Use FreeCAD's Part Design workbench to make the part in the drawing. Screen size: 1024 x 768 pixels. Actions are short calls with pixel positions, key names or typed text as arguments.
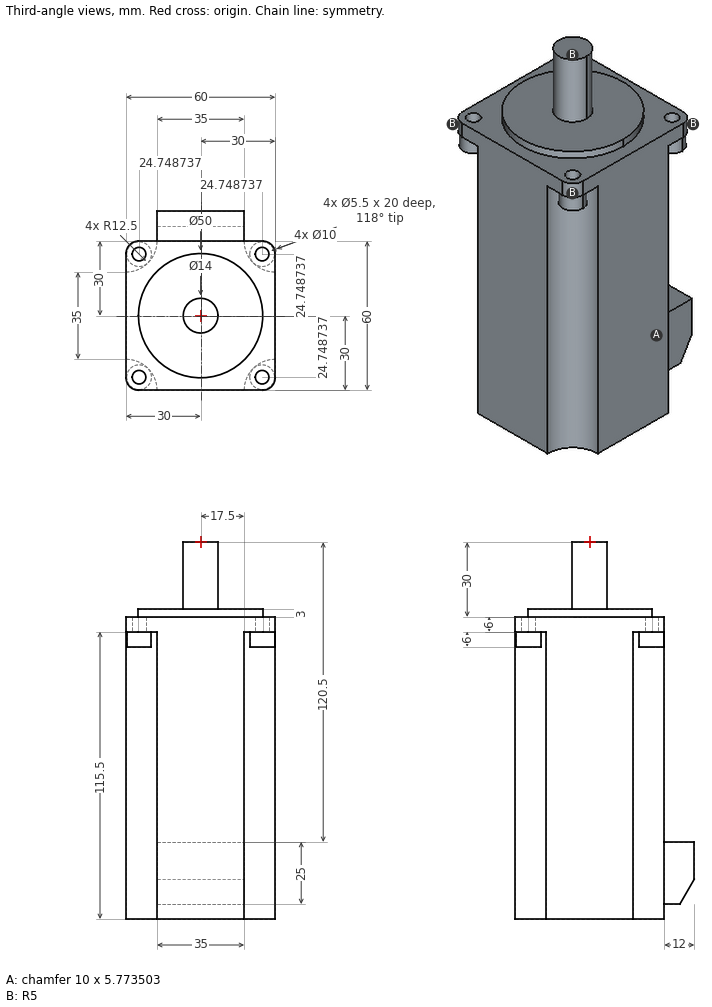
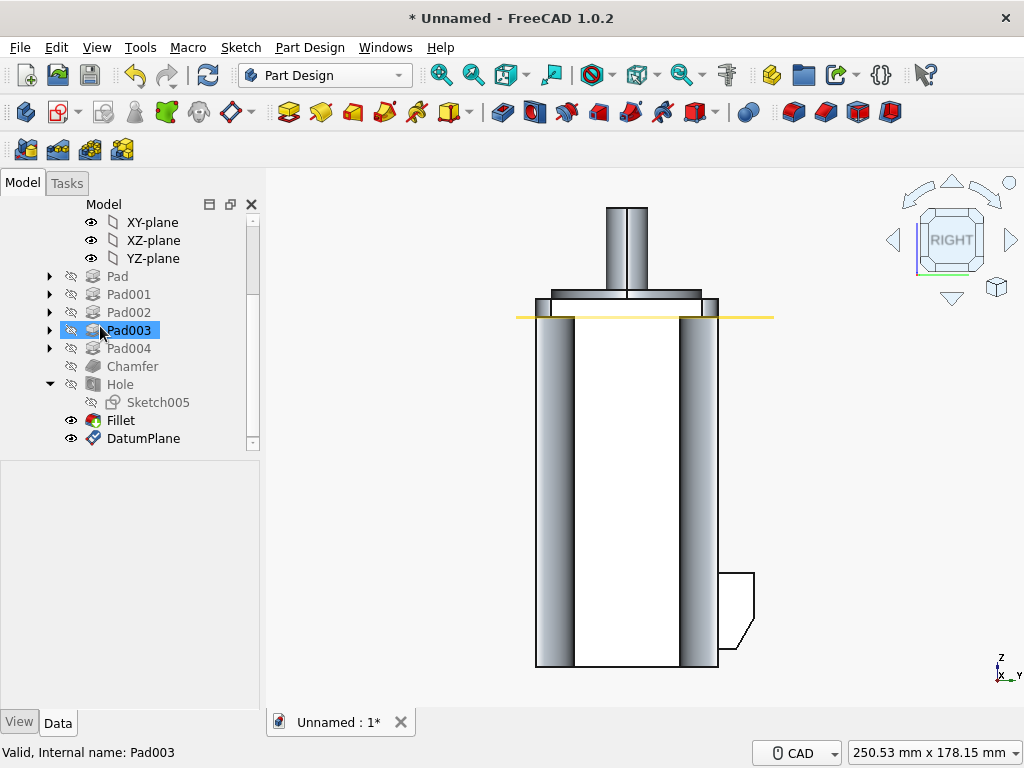
click(116, 438)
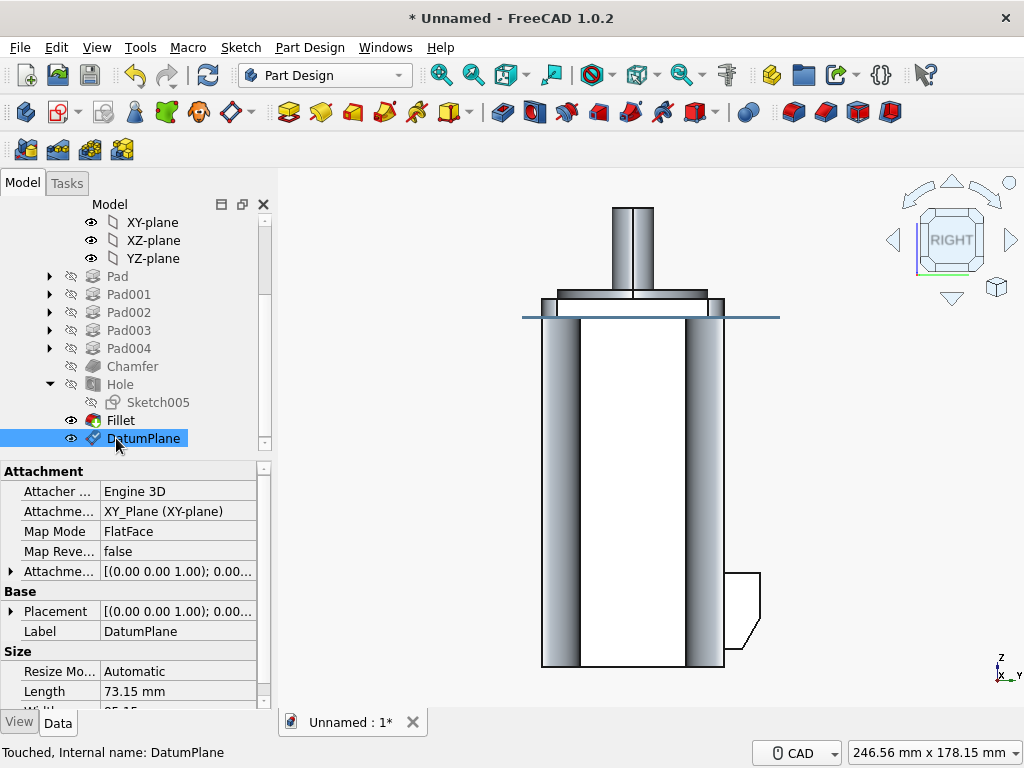
click(58, 112)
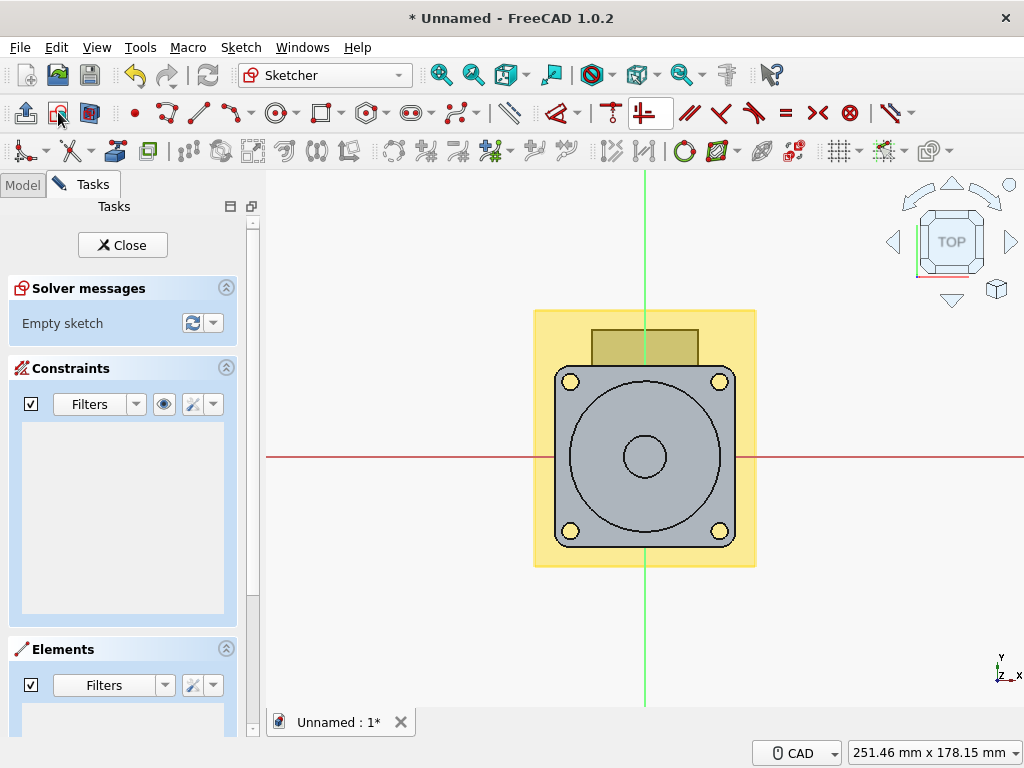
click(90, 114)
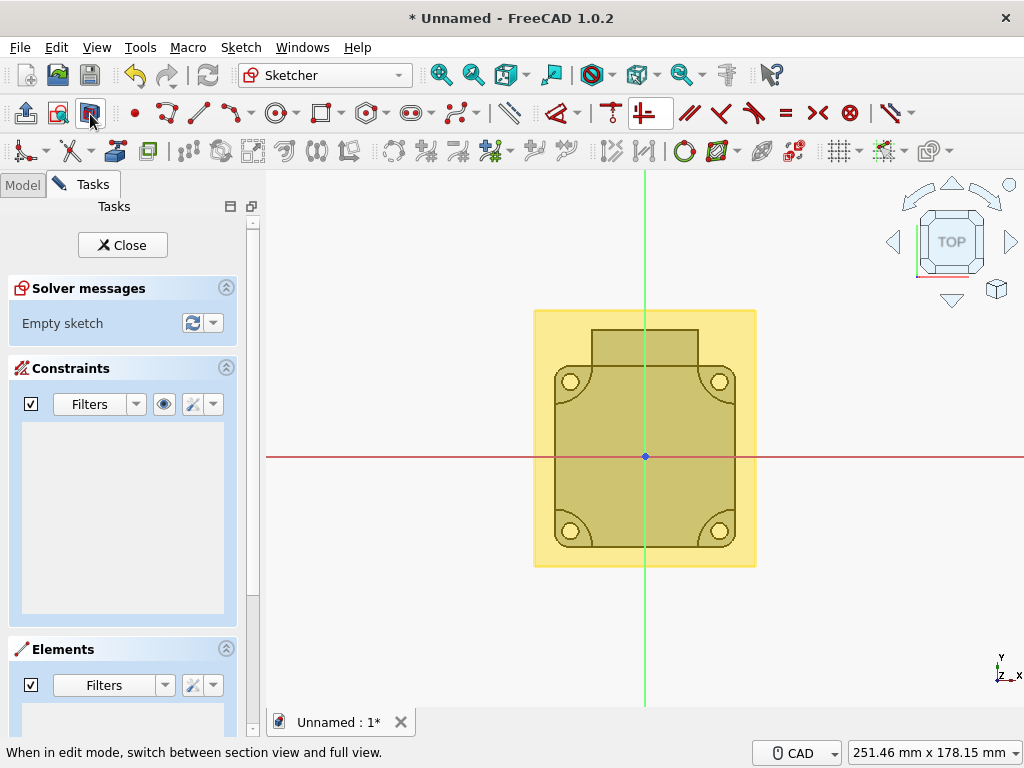
scroll(728, 479, up, 3)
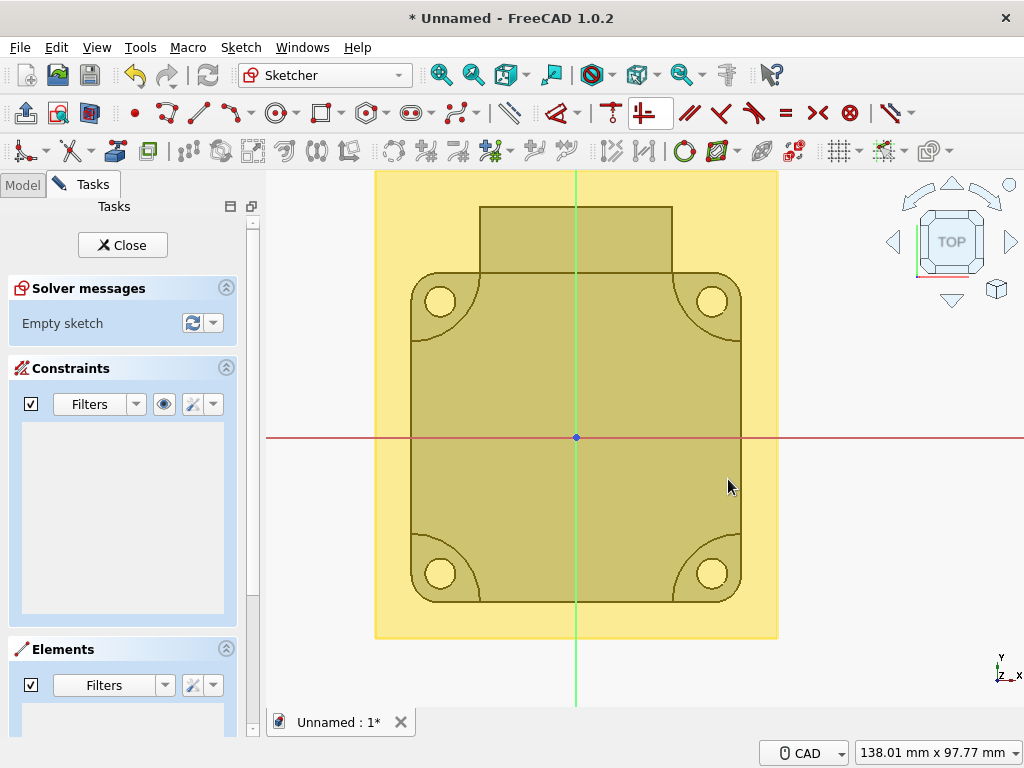
click(276, 114)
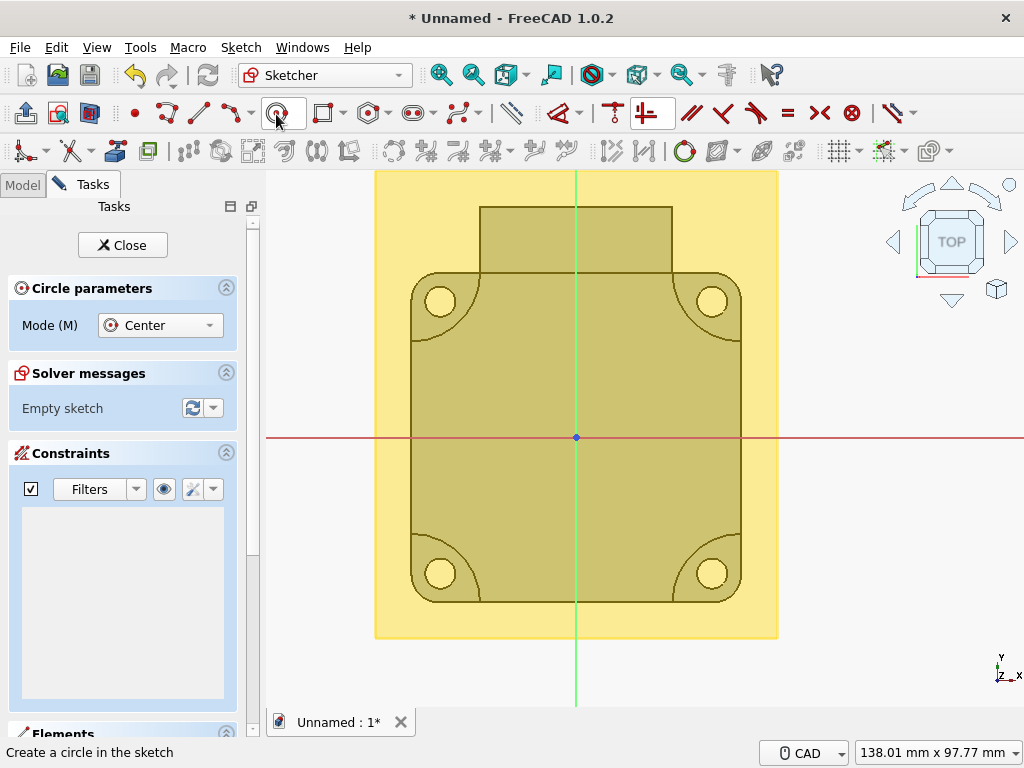
click(712, 302)
click(732, 282)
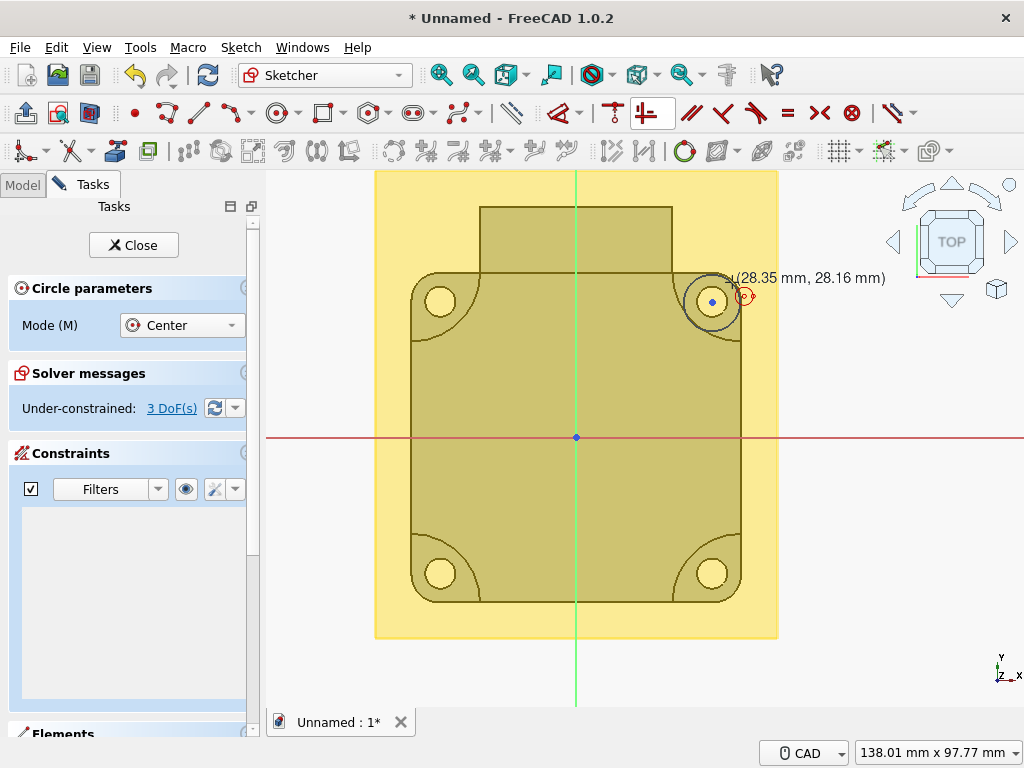
click(712, 574)
click(732, 554)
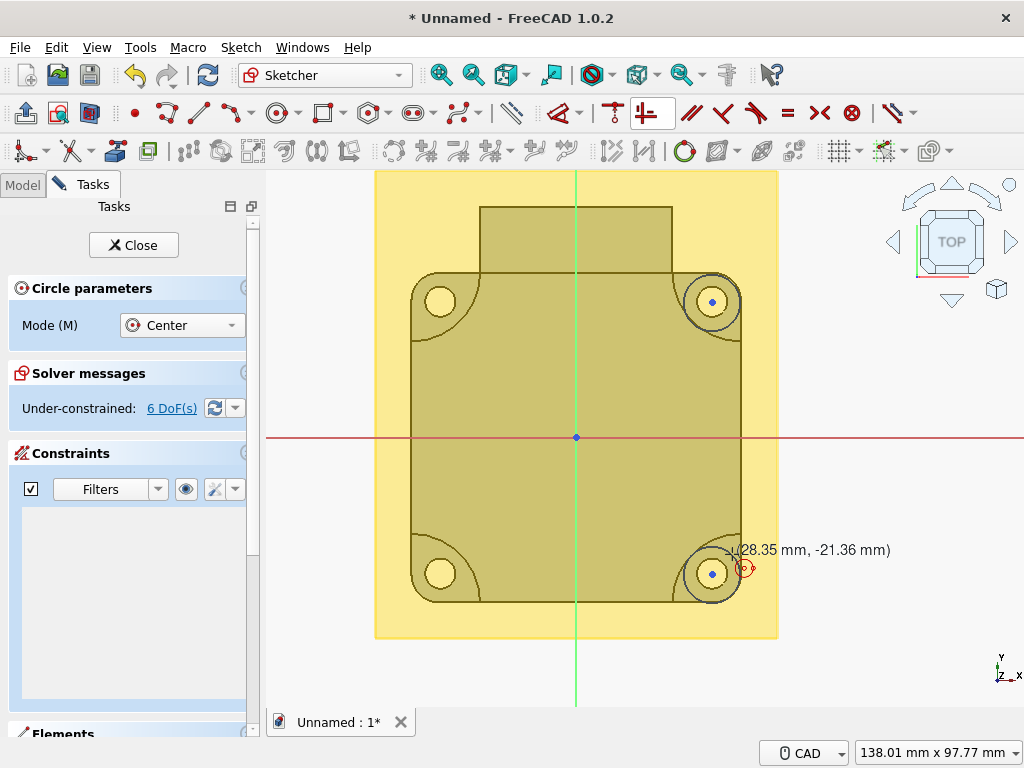
click(440, 574)
click(460, 554)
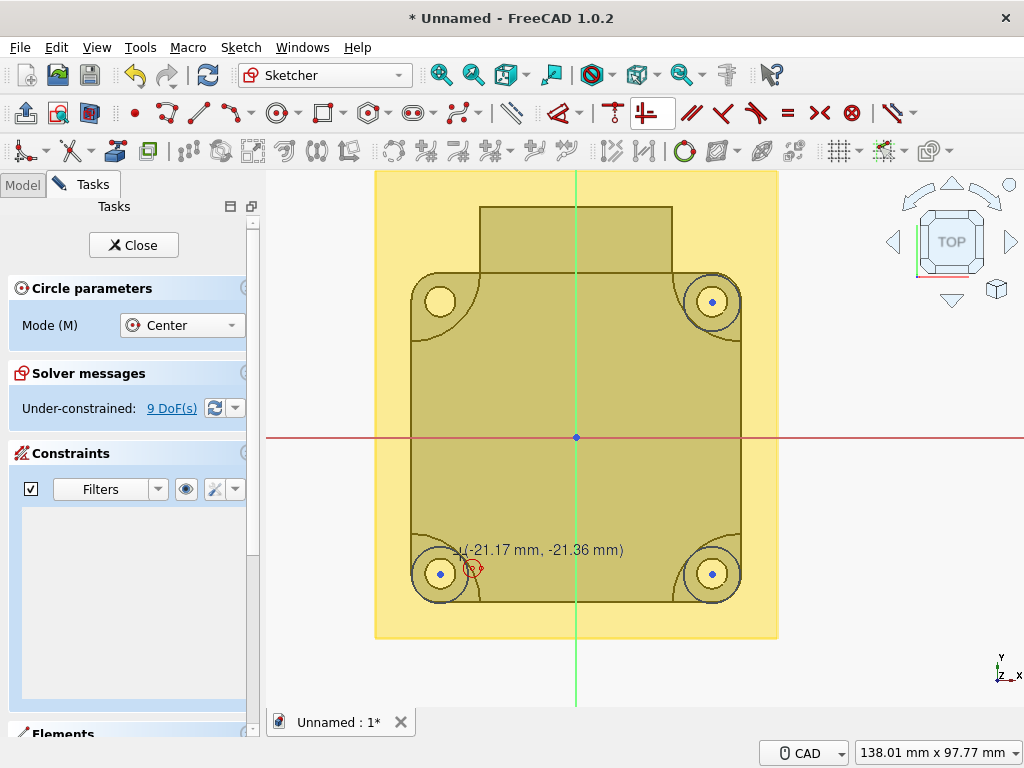
click(440, 302)
click(460, 282)
key(Escape)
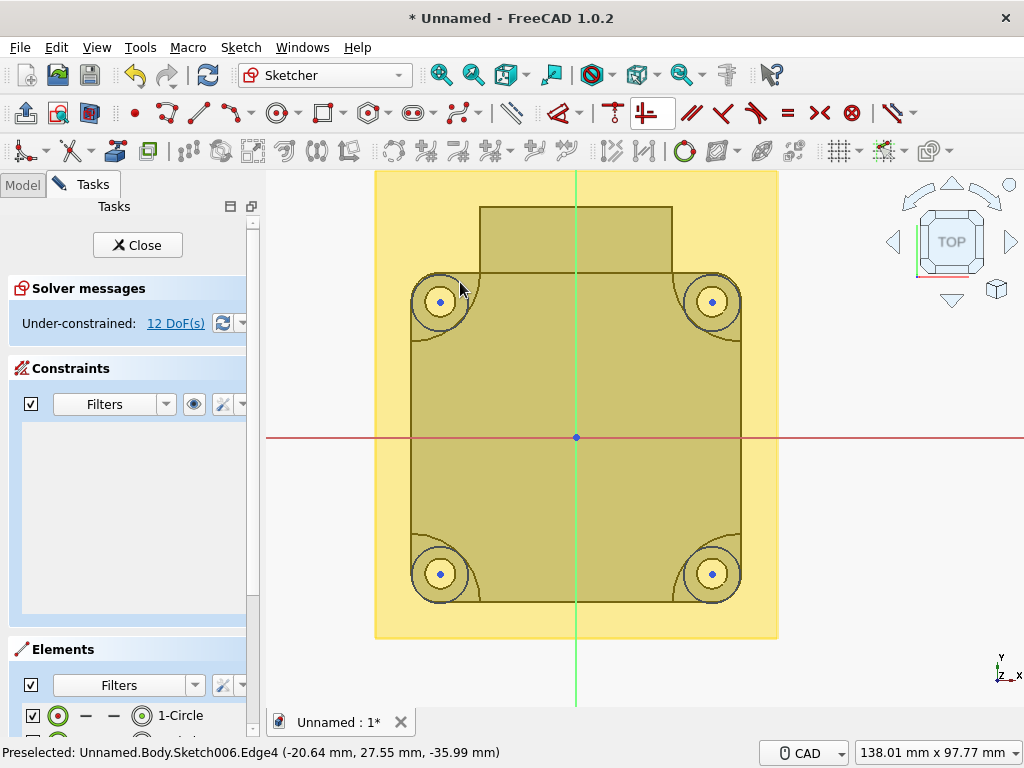
click(732, 283)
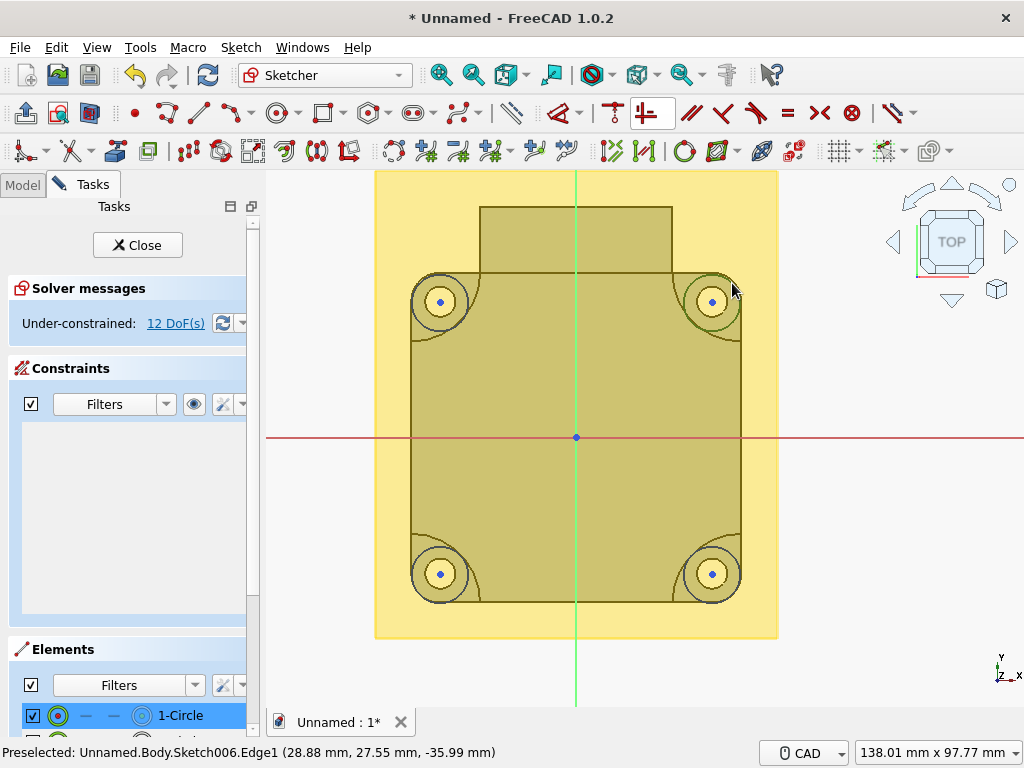
click(732, 555)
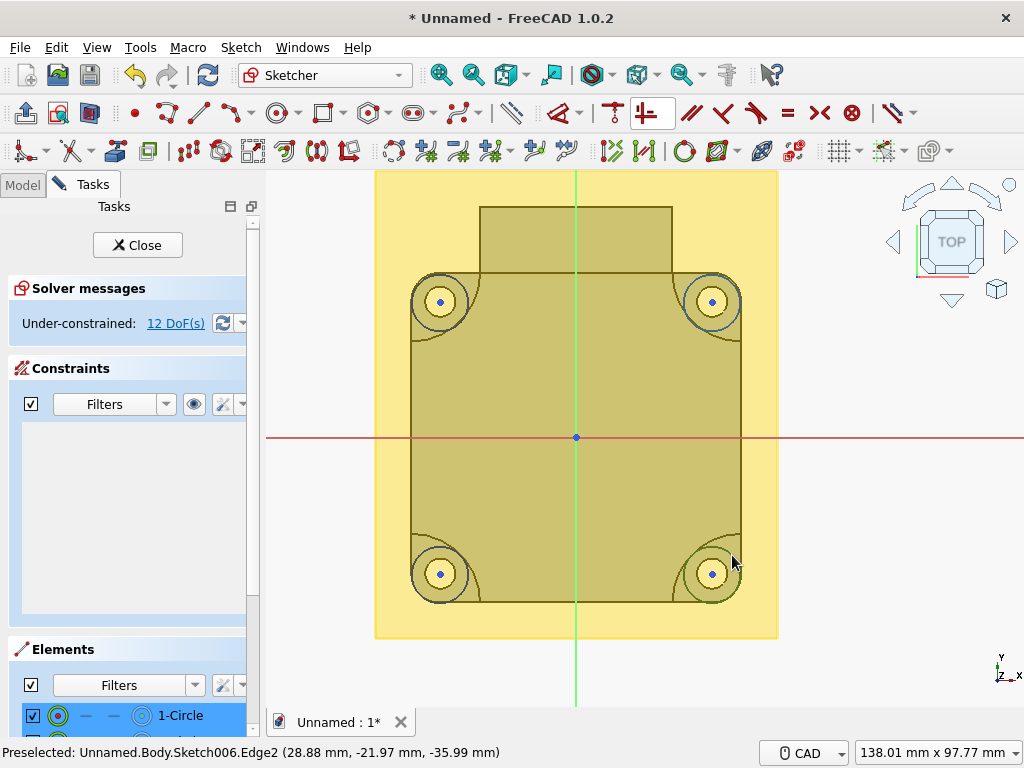
click(460, 555)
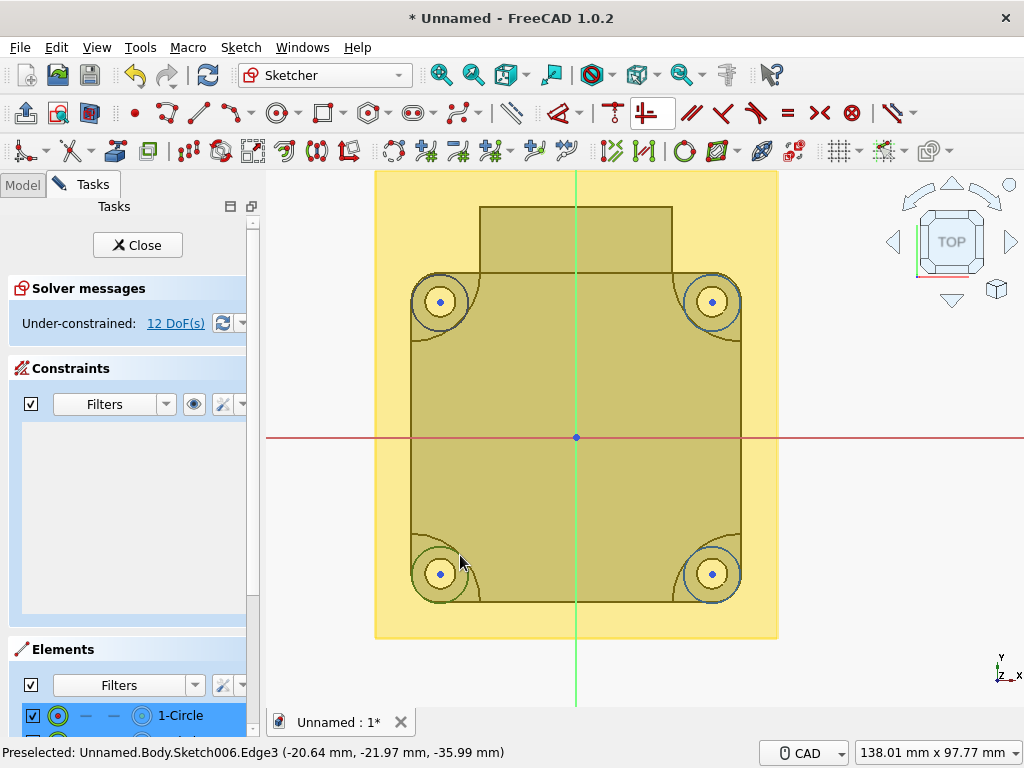
click(460, 283)